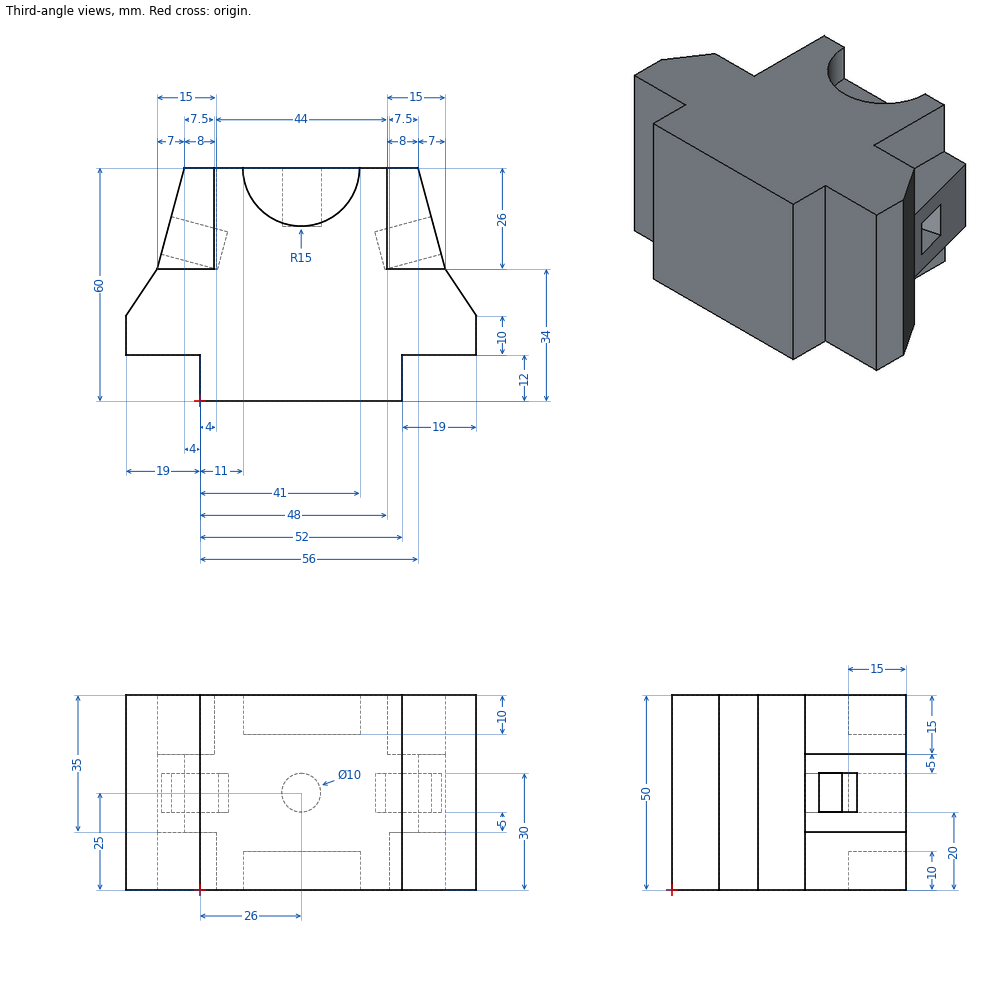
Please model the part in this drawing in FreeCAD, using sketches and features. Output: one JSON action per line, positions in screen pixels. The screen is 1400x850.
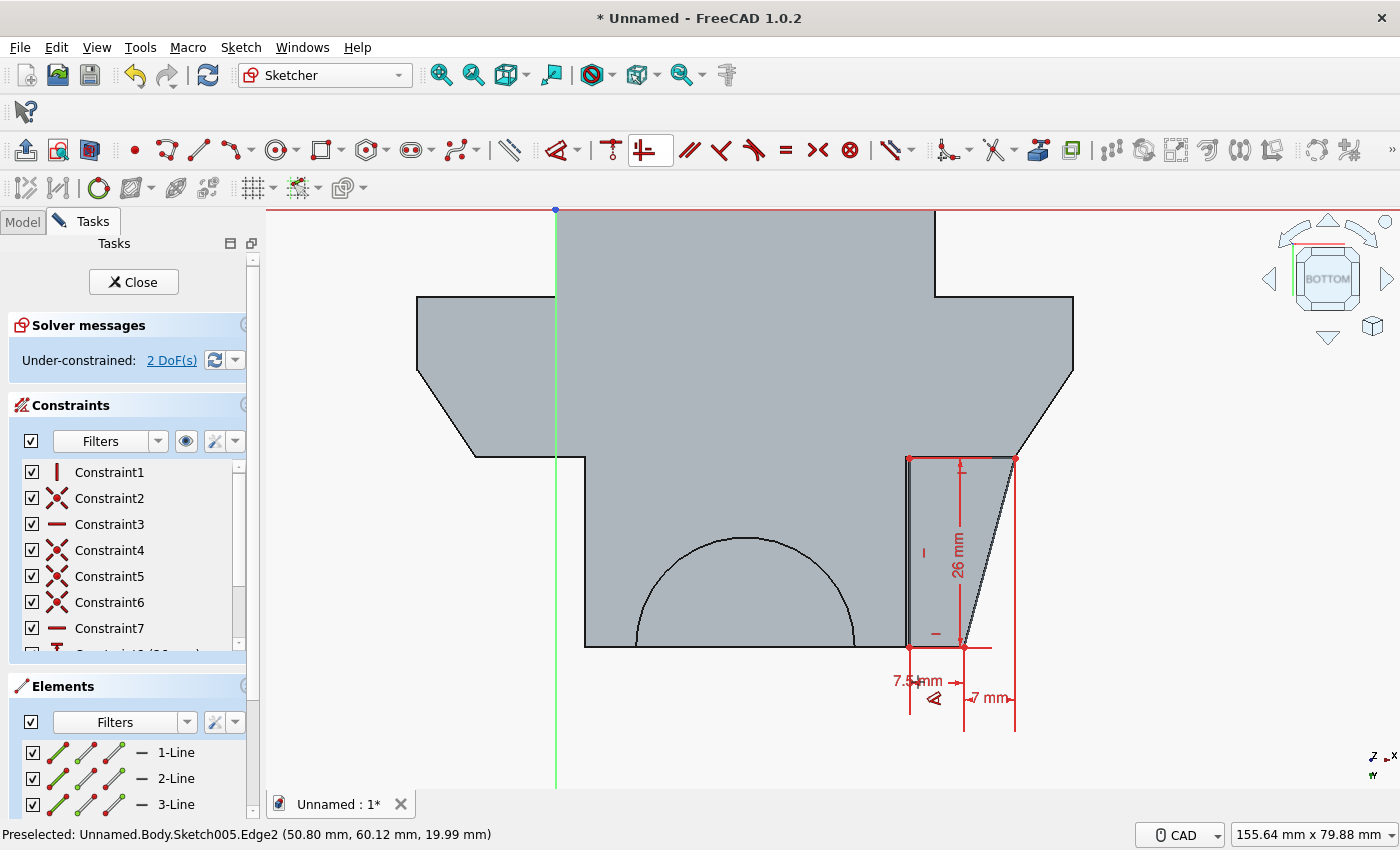
{"action": "left_click", "coordinate": [910, 458]}
{"action": "left_click", "coordinate": [522, 347]}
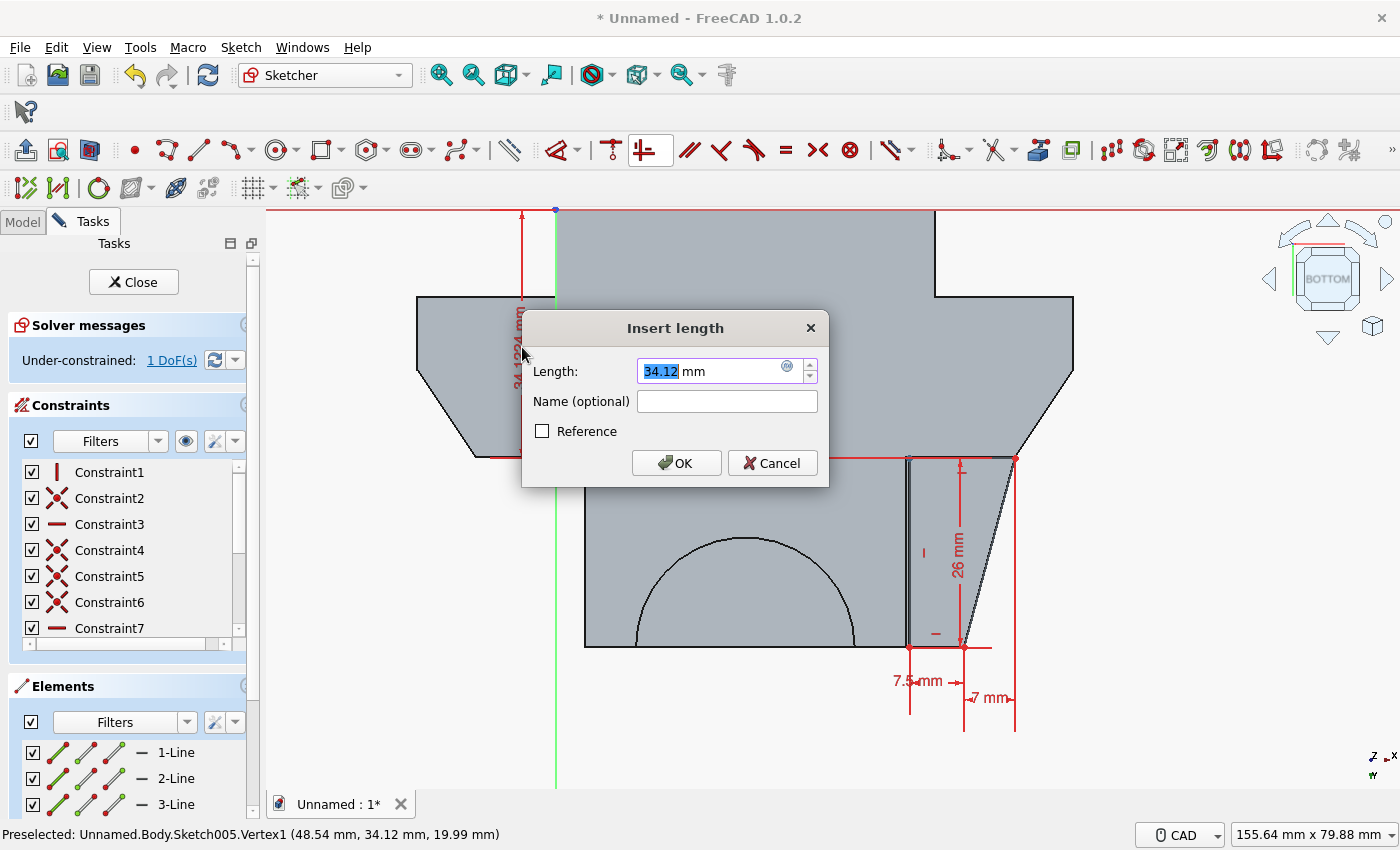
{"action": "type", "text": "34"}
{"action": "key", "text": "Return"}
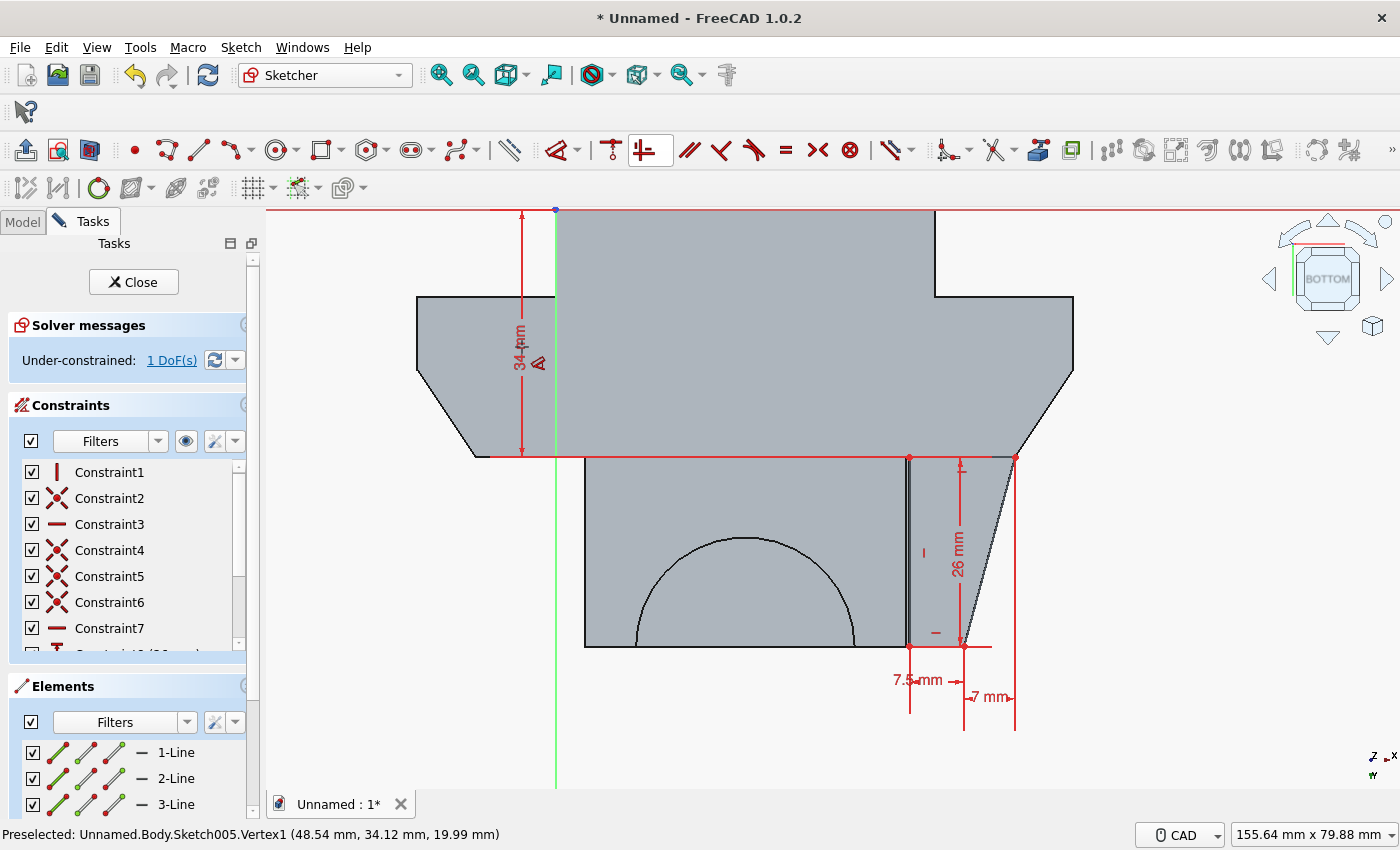
{"action": "left_click", "coordinate": [964, 647]}
{"action": "left_click", "coordinate": [760, 681]}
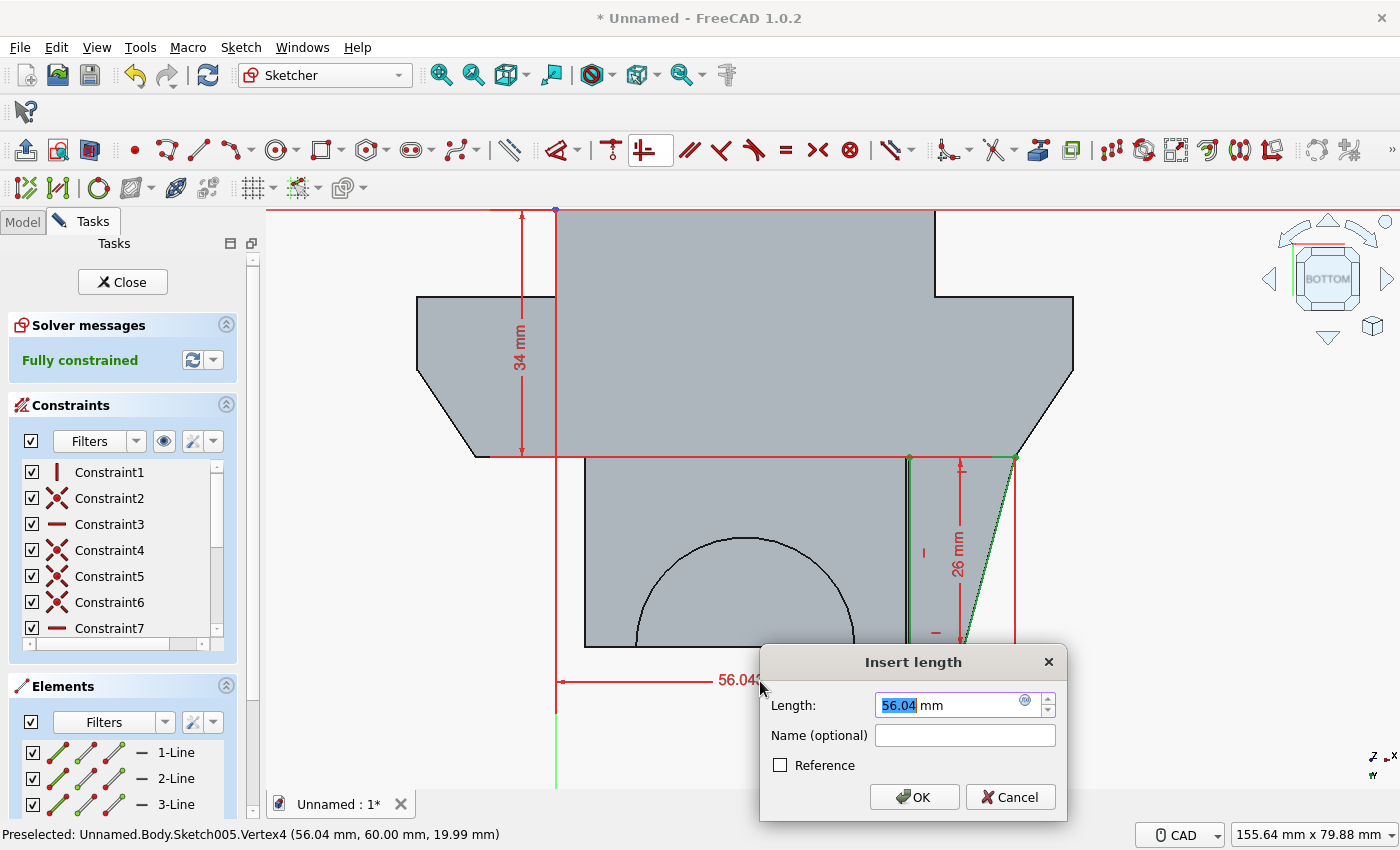
{"action": "type", "text": "56"}
{"action": "key", "text": "Return"}
{"action": "key", "text": "Escape"}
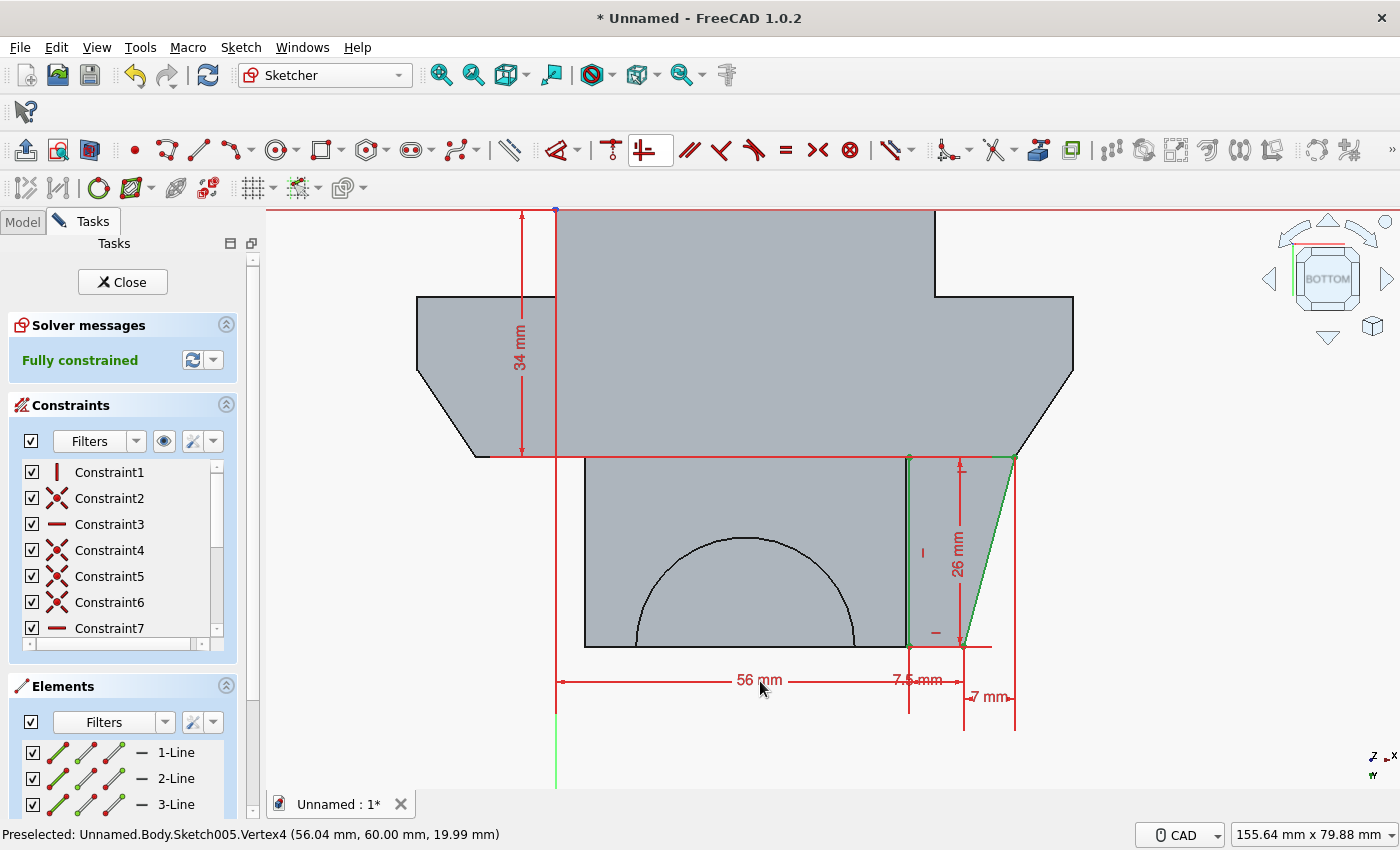
{"action": "left_click", "coordinate": [123, 282]}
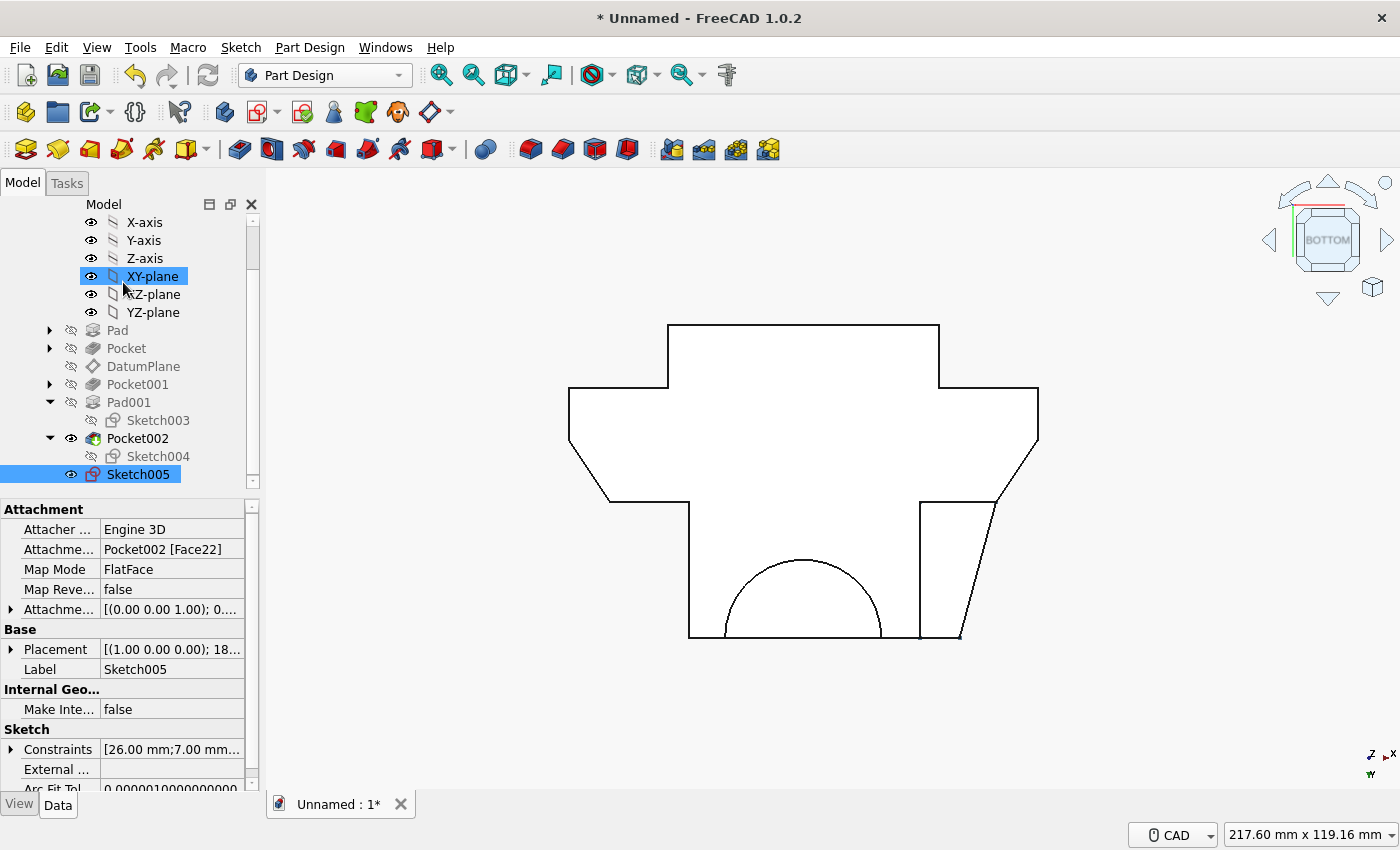
{"action": "left_click", "coordinate": [26, 150]}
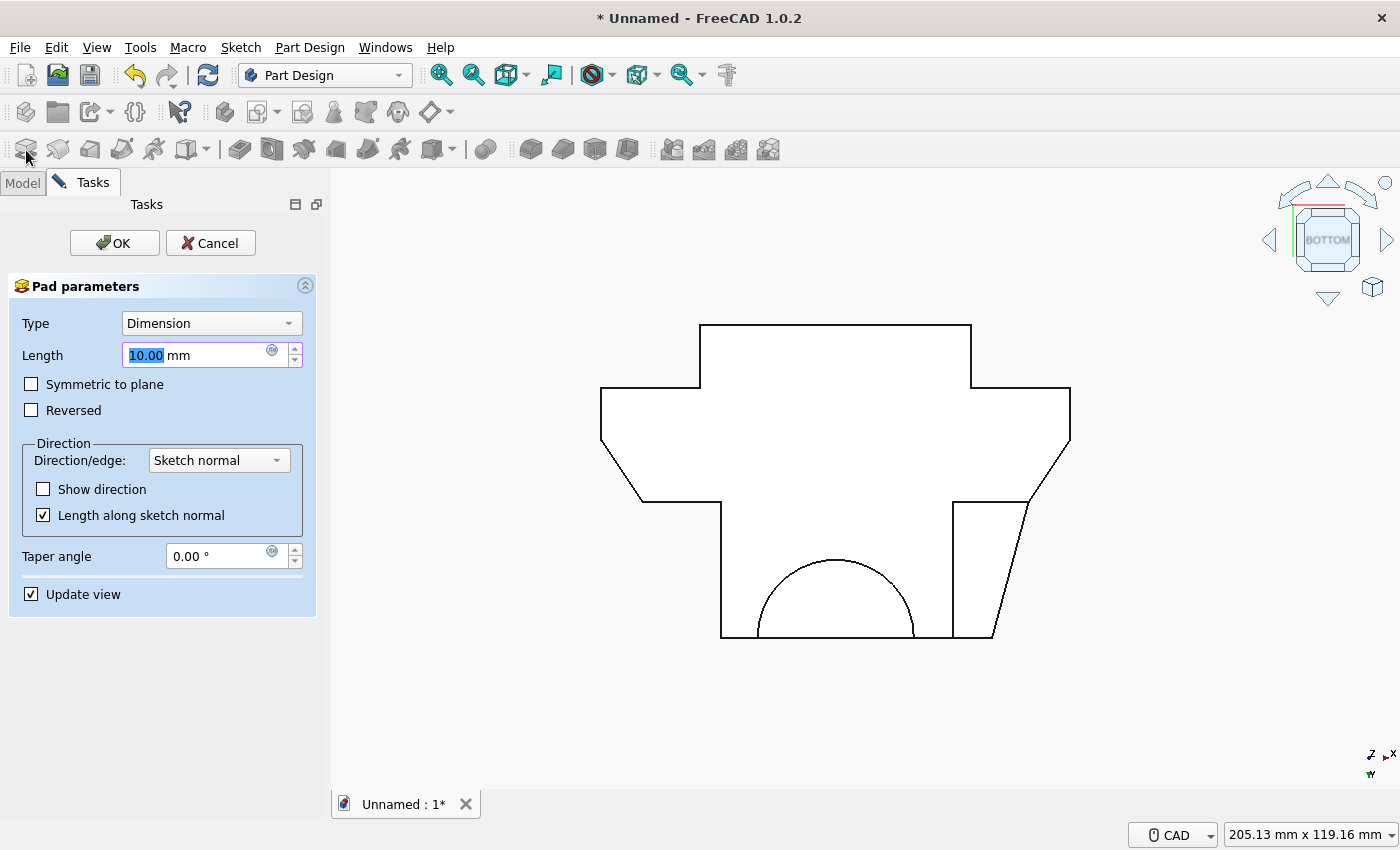
{"action": "type", "text": "5"}
{"action": "key", "text": "Tab"}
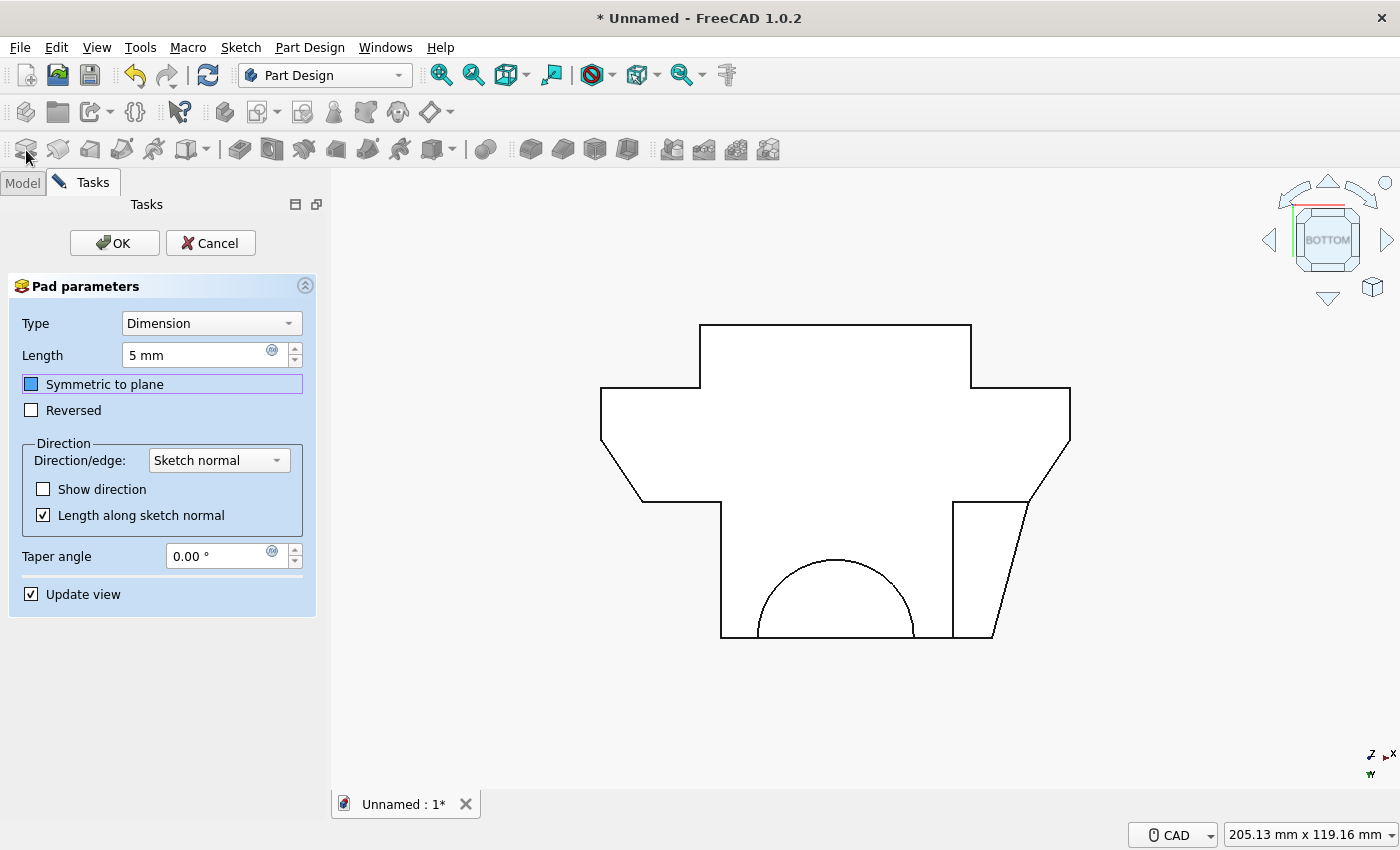
{"action": "left_click", "coordinate": [115, 243]}